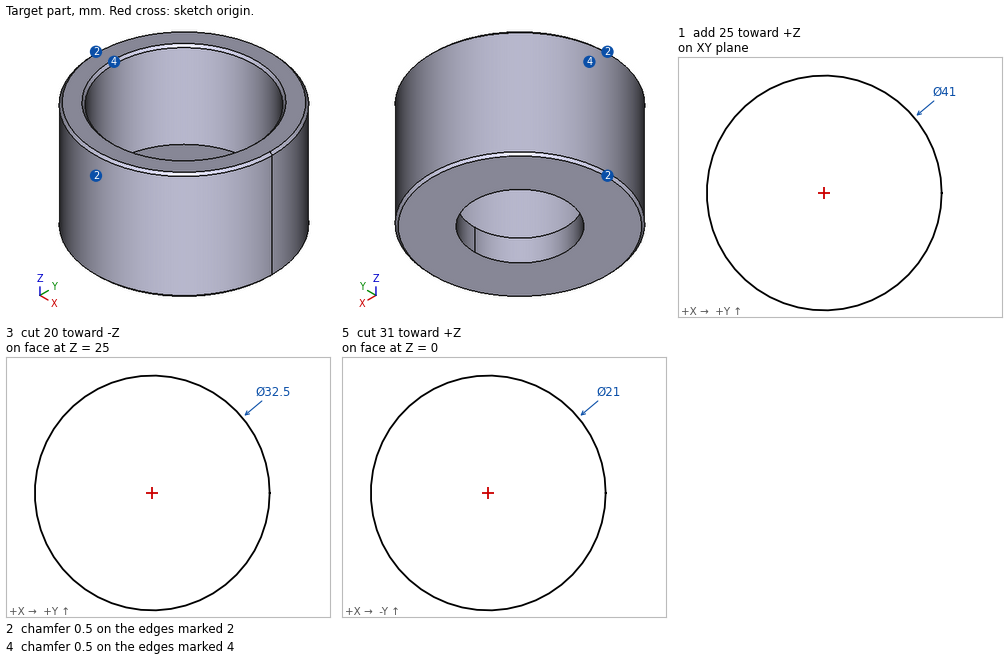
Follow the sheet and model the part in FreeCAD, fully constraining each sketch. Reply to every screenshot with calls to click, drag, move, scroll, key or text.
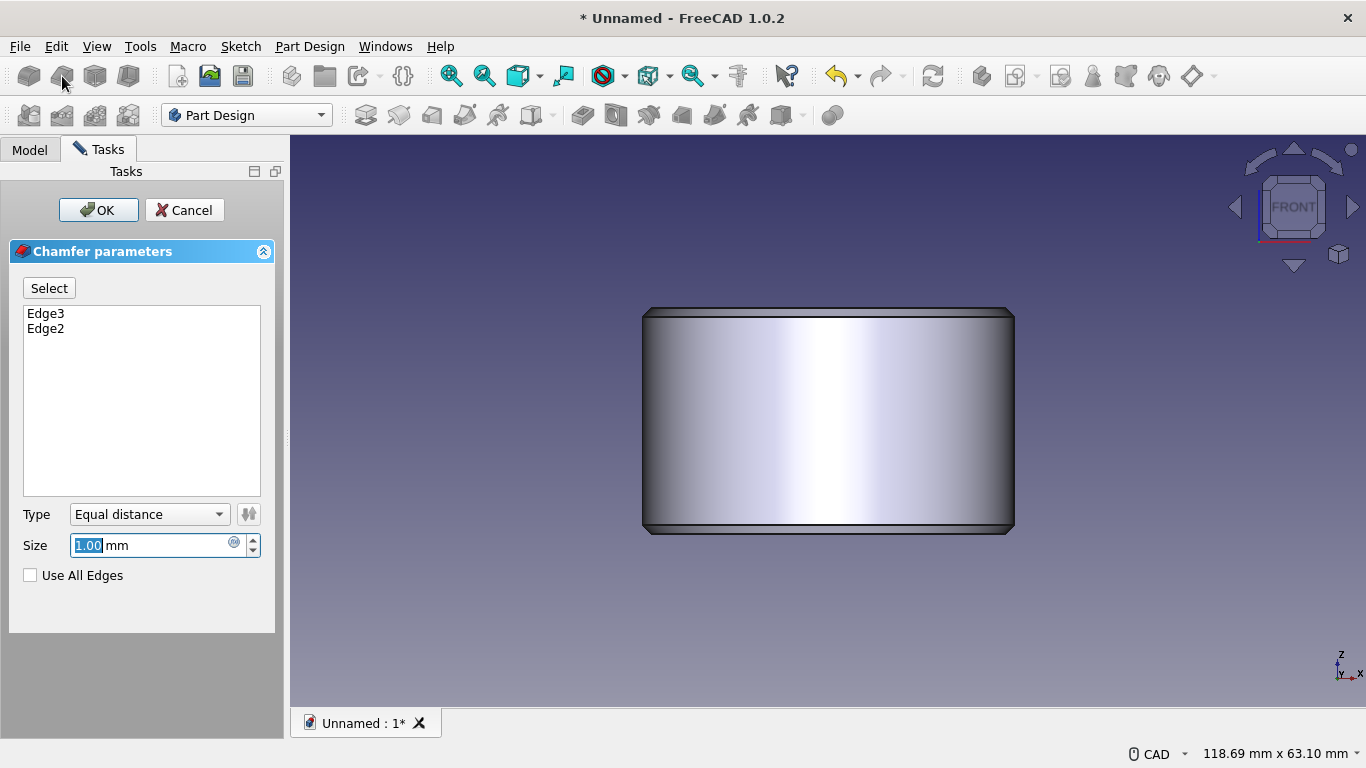
text(0.5)
key(Tab)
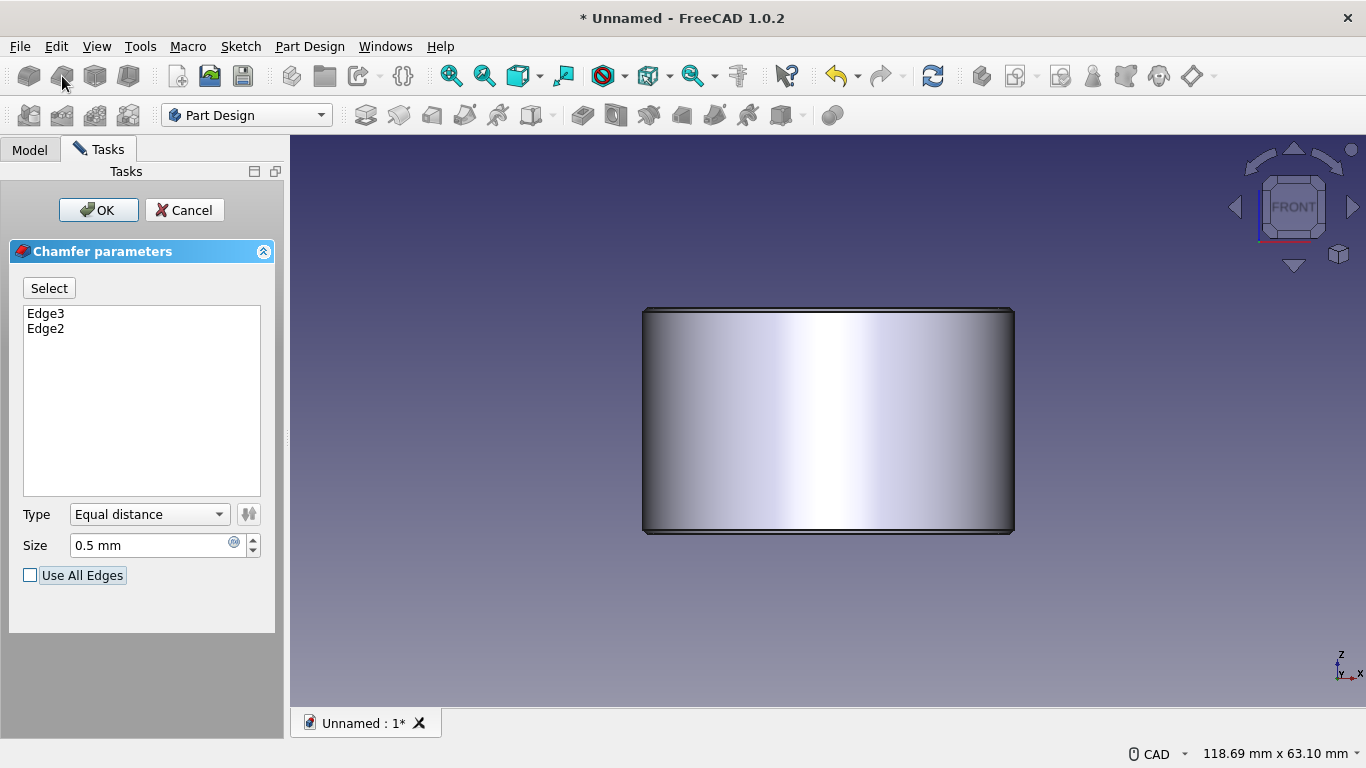
click(99, 210)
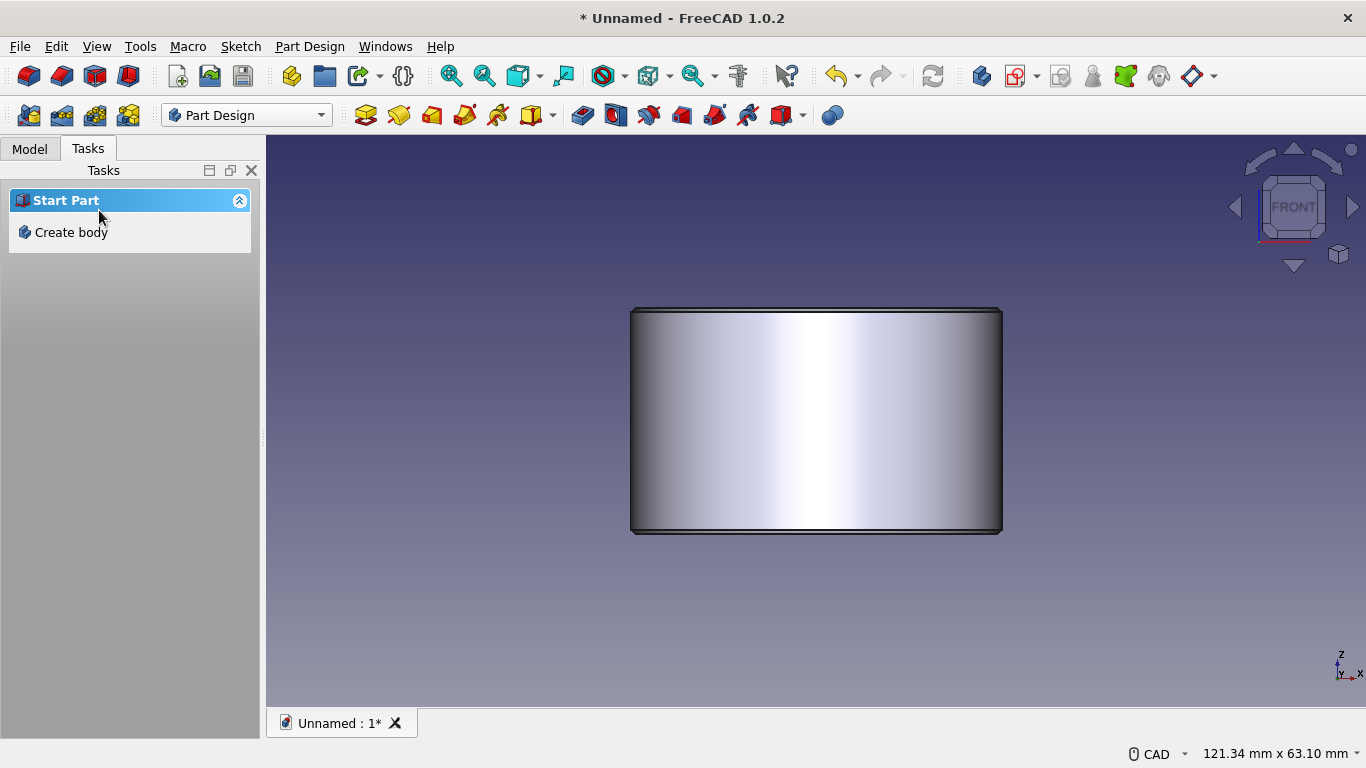
click(452, 76)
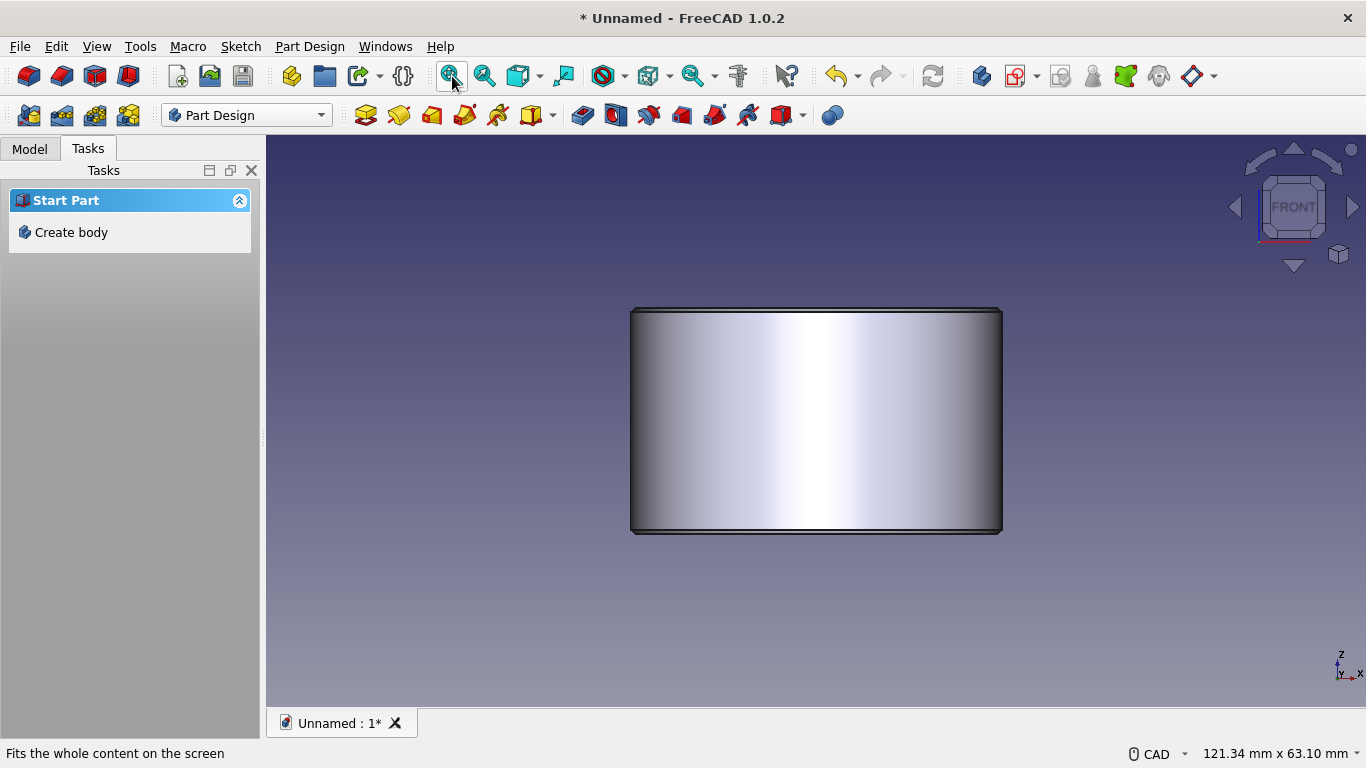
key(0)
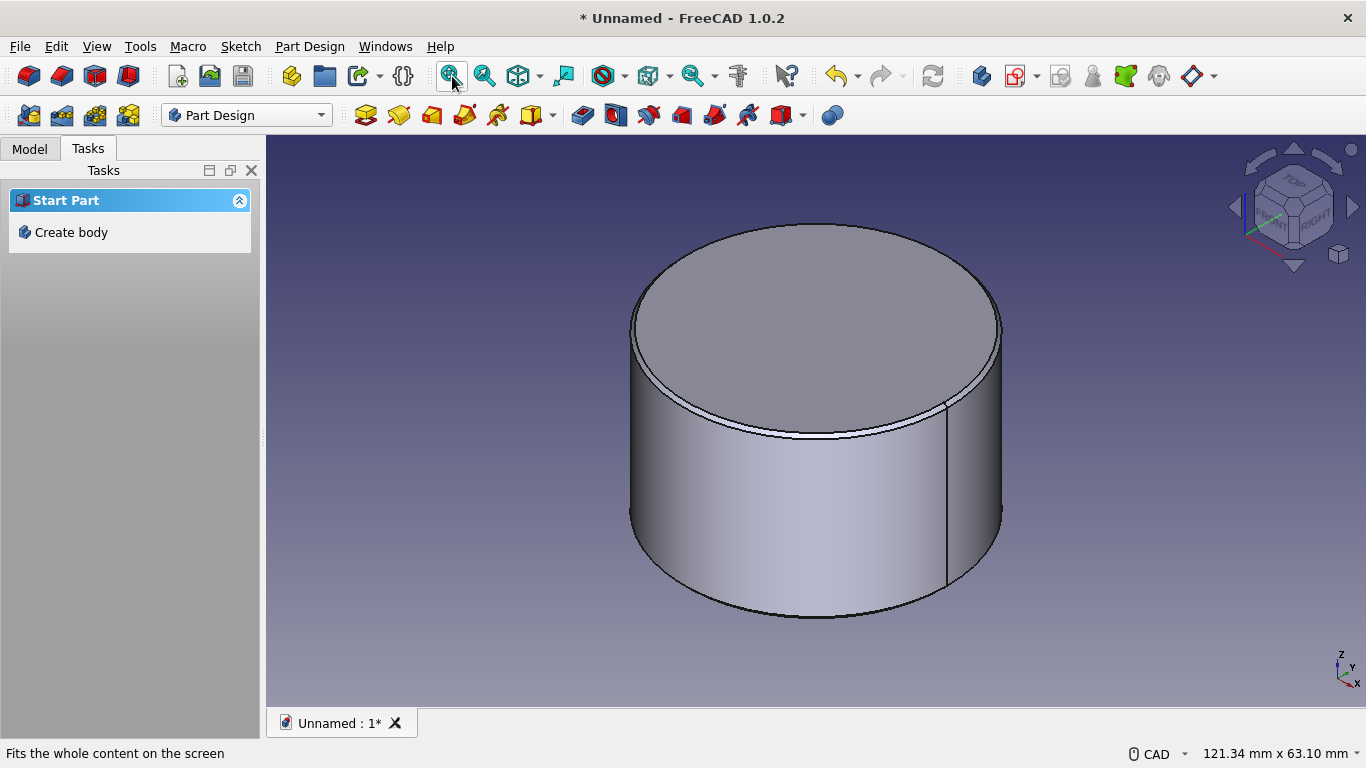
click(816, 327)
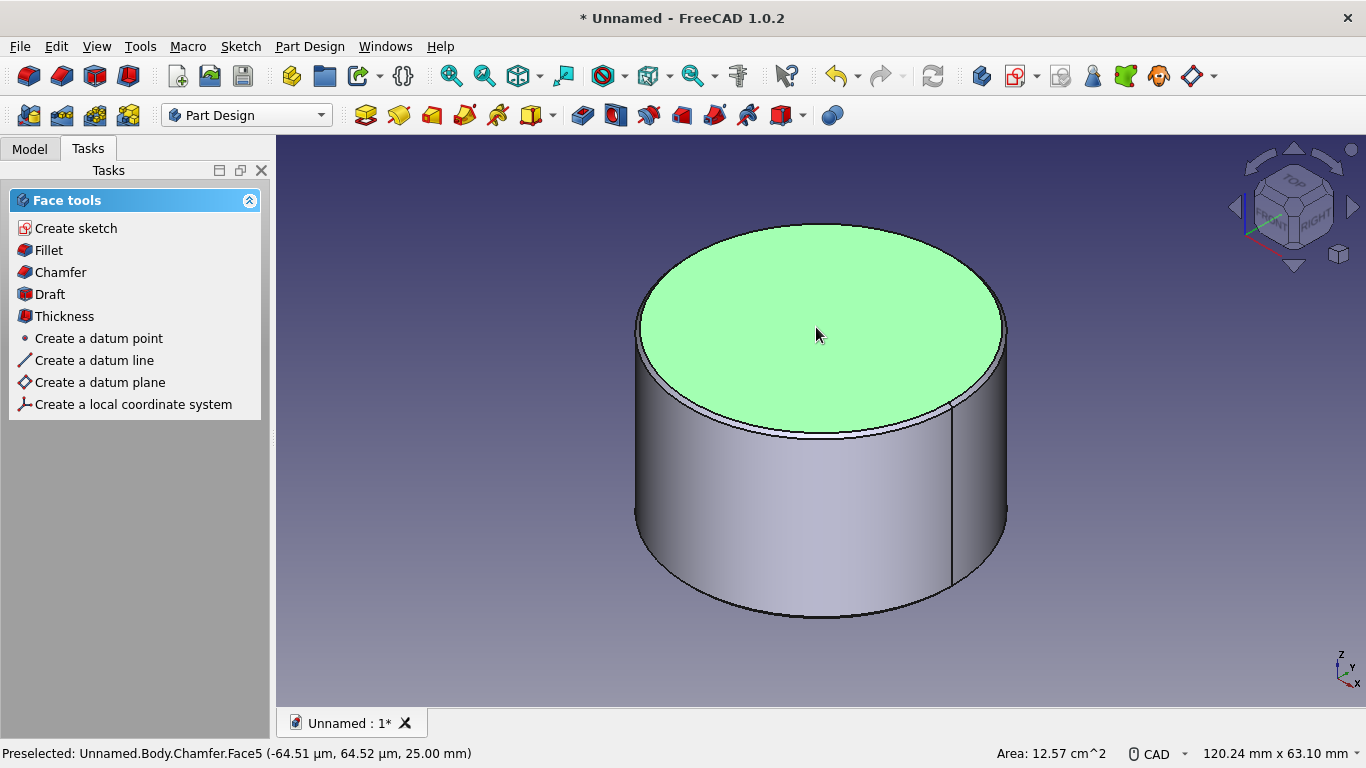
click(1014, 76)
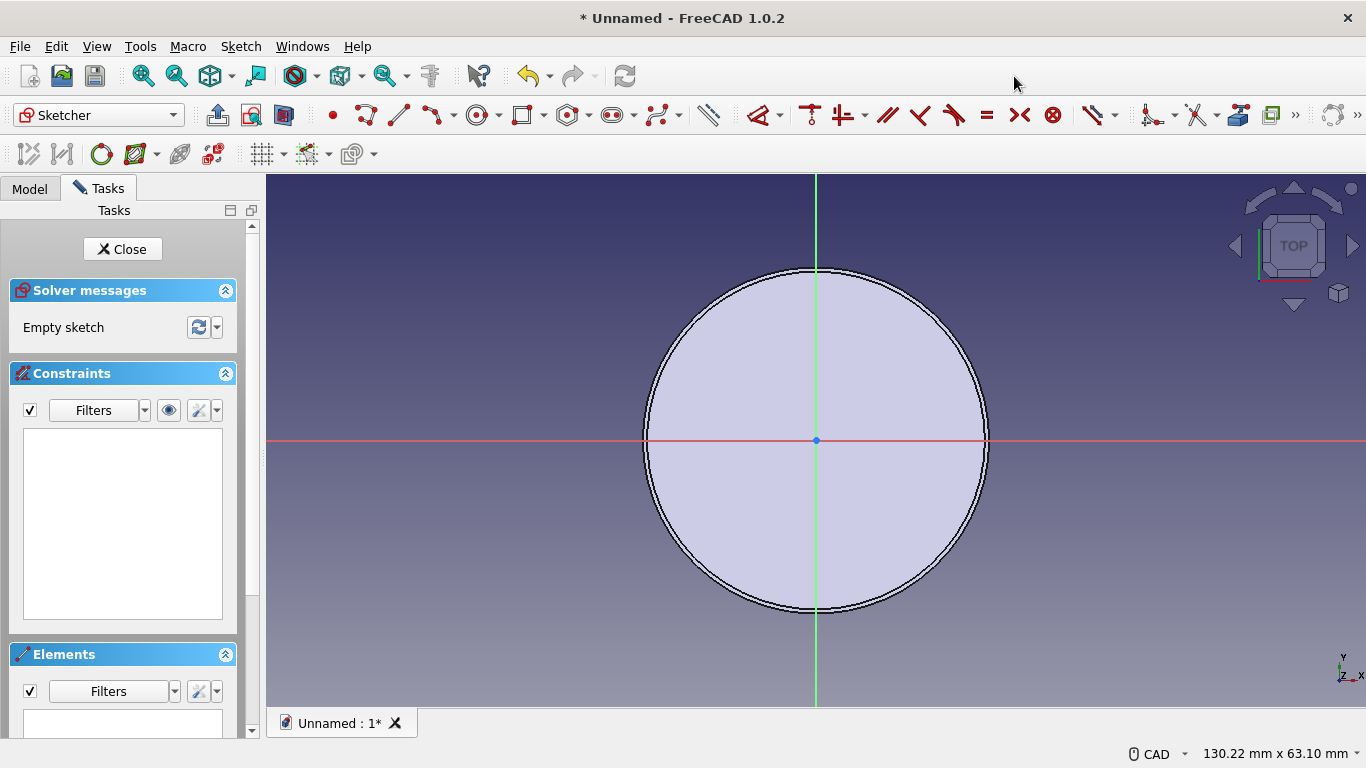
click(476, 116)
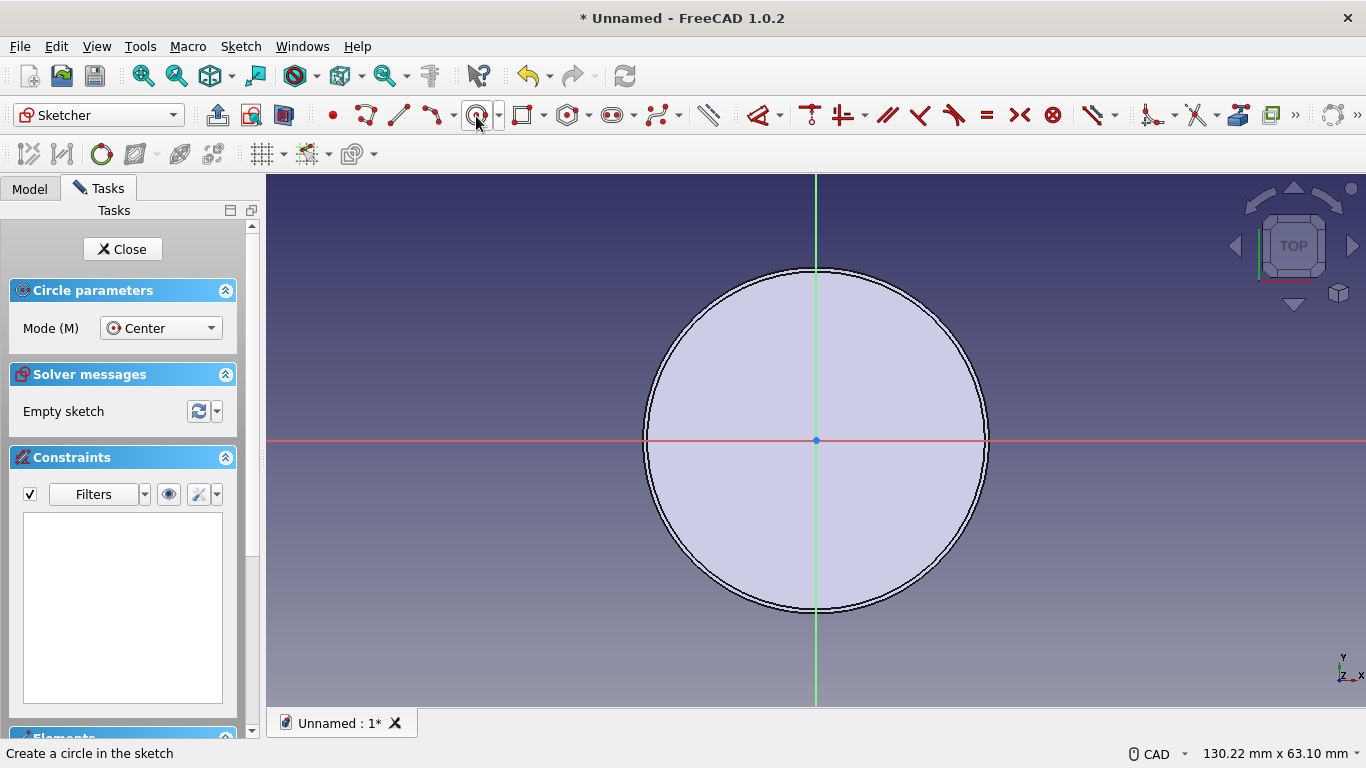
click(816, 441)
move(913, 343)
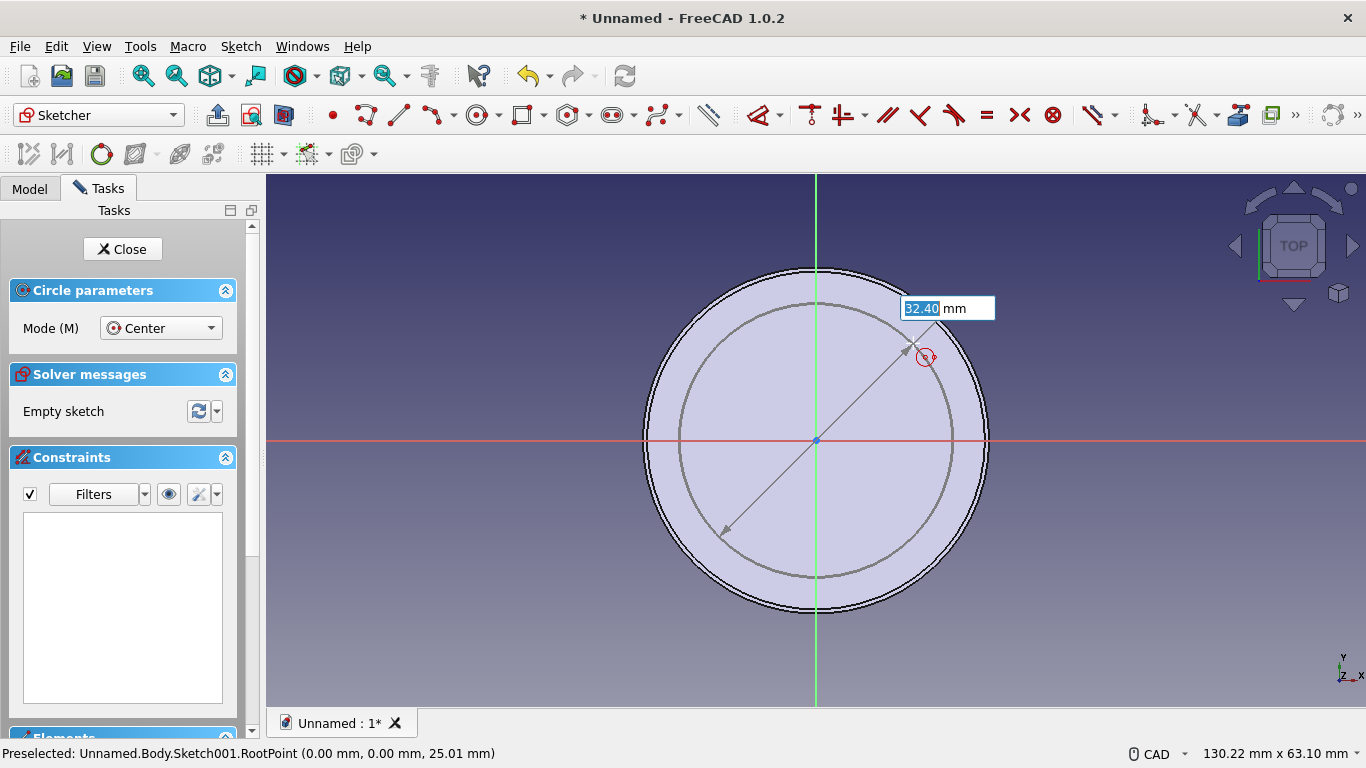
text(32.5)
key(Return)
key(Escape)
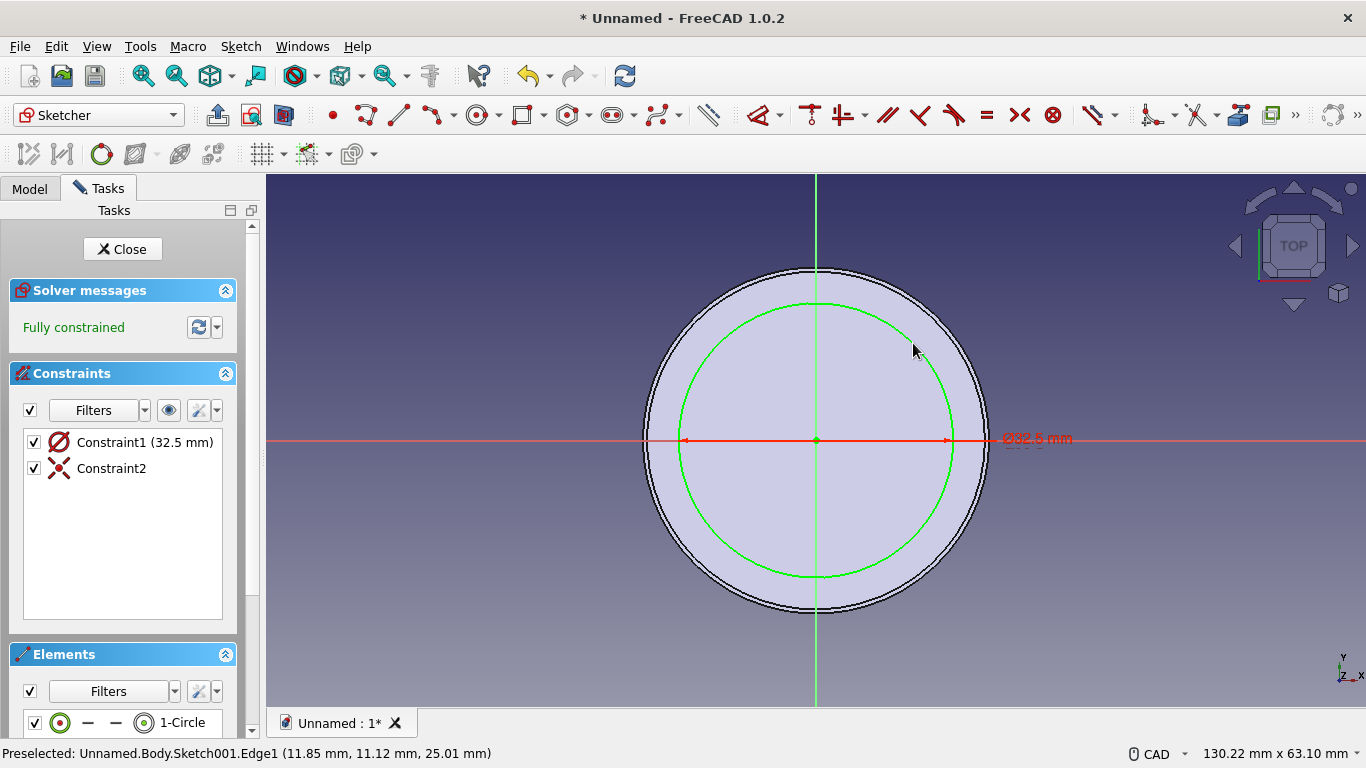
click(123, 249)